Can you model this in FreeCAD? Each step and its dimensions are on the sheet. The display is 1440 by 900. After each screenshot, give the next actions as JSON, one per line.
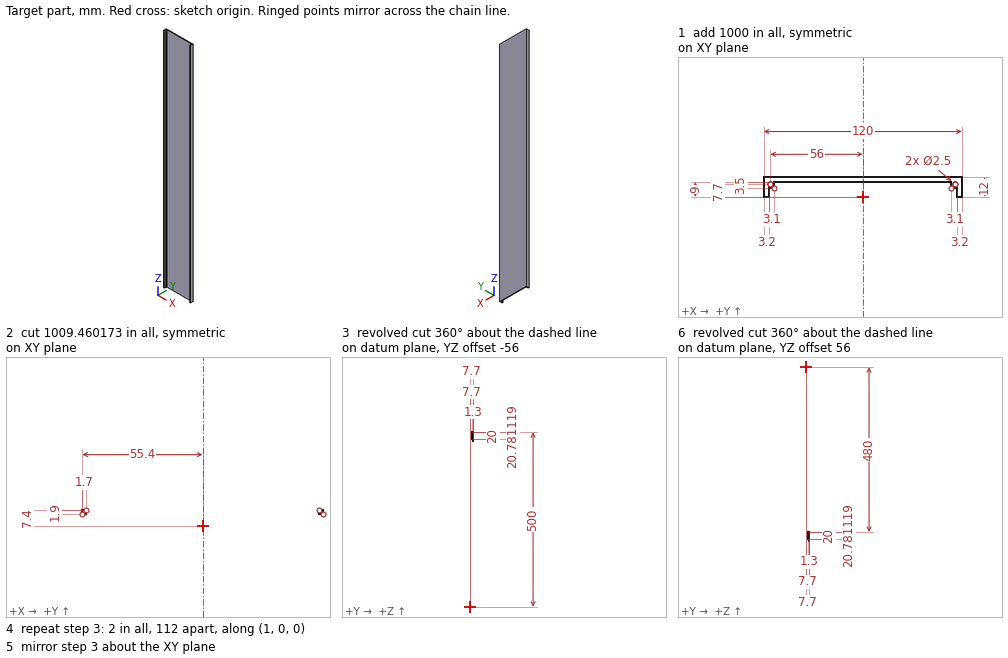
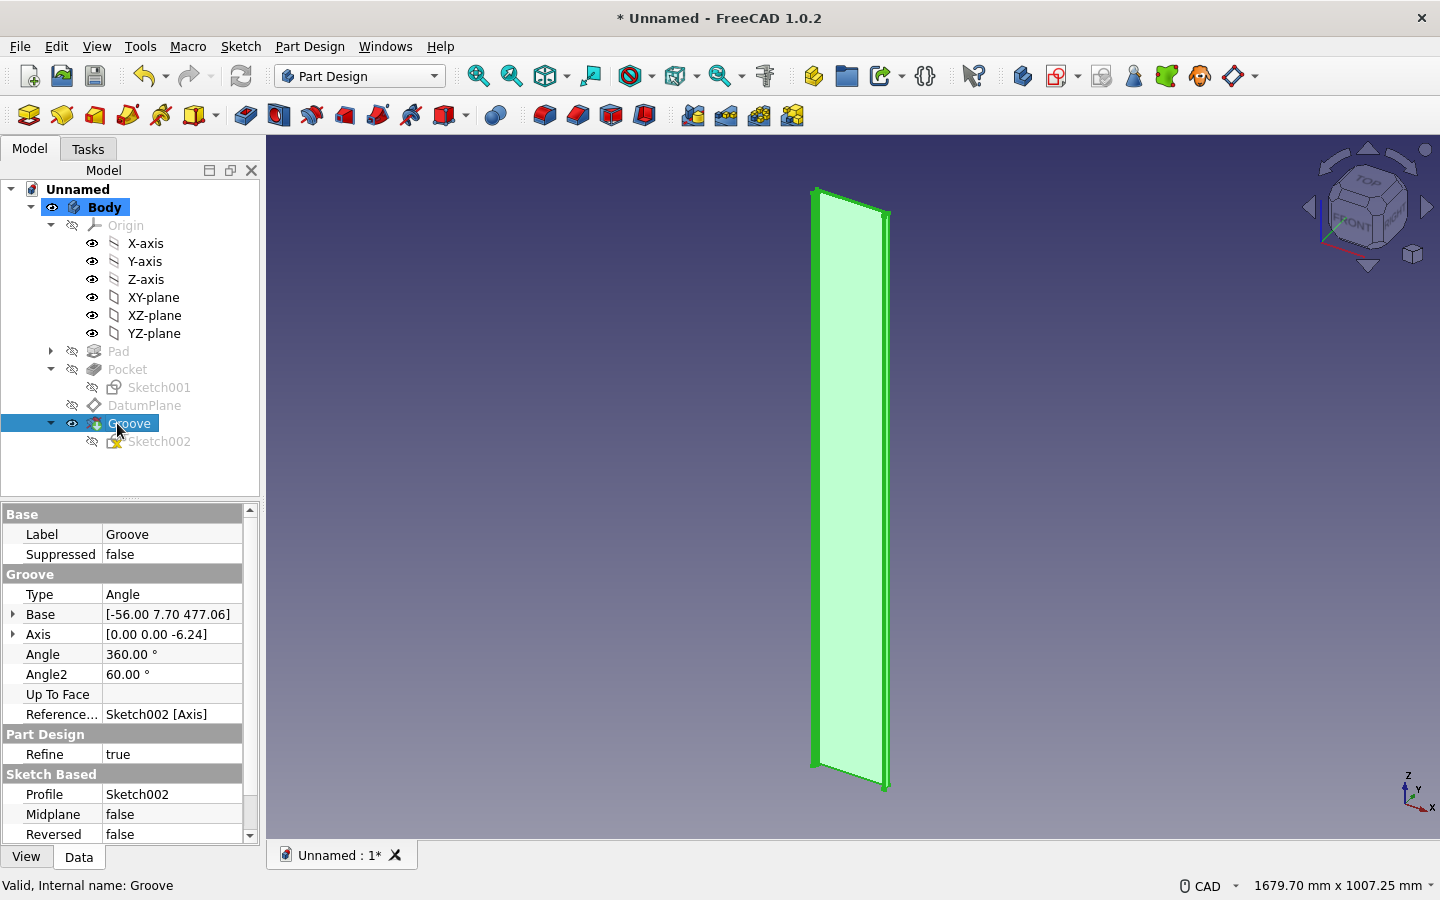
{"action": "left_click", "coordinate": [726, 116]}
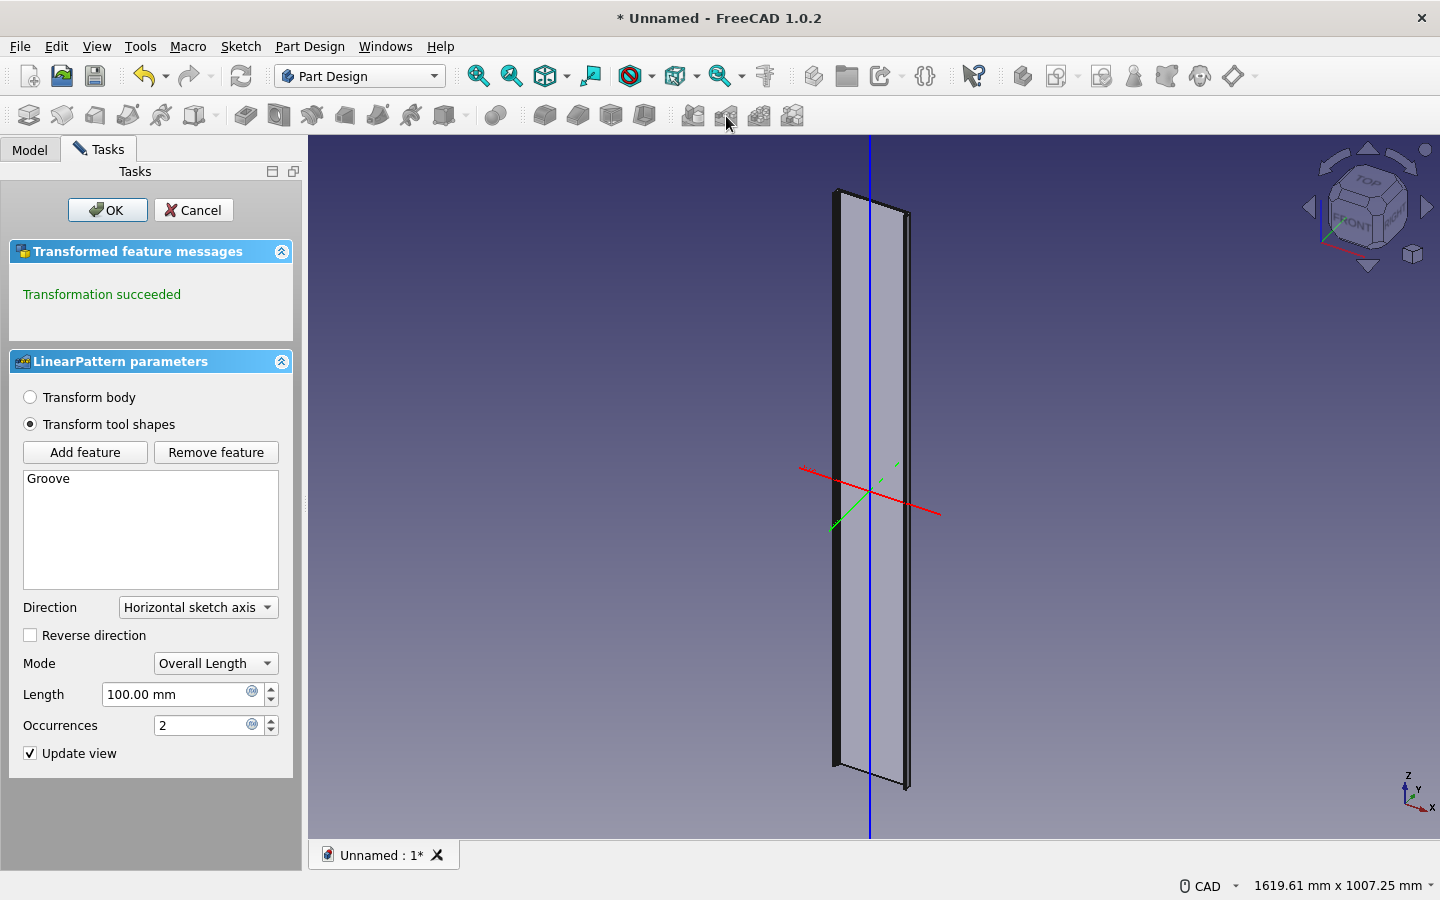
{"action": "left_click", "coordinate": [199, 608]}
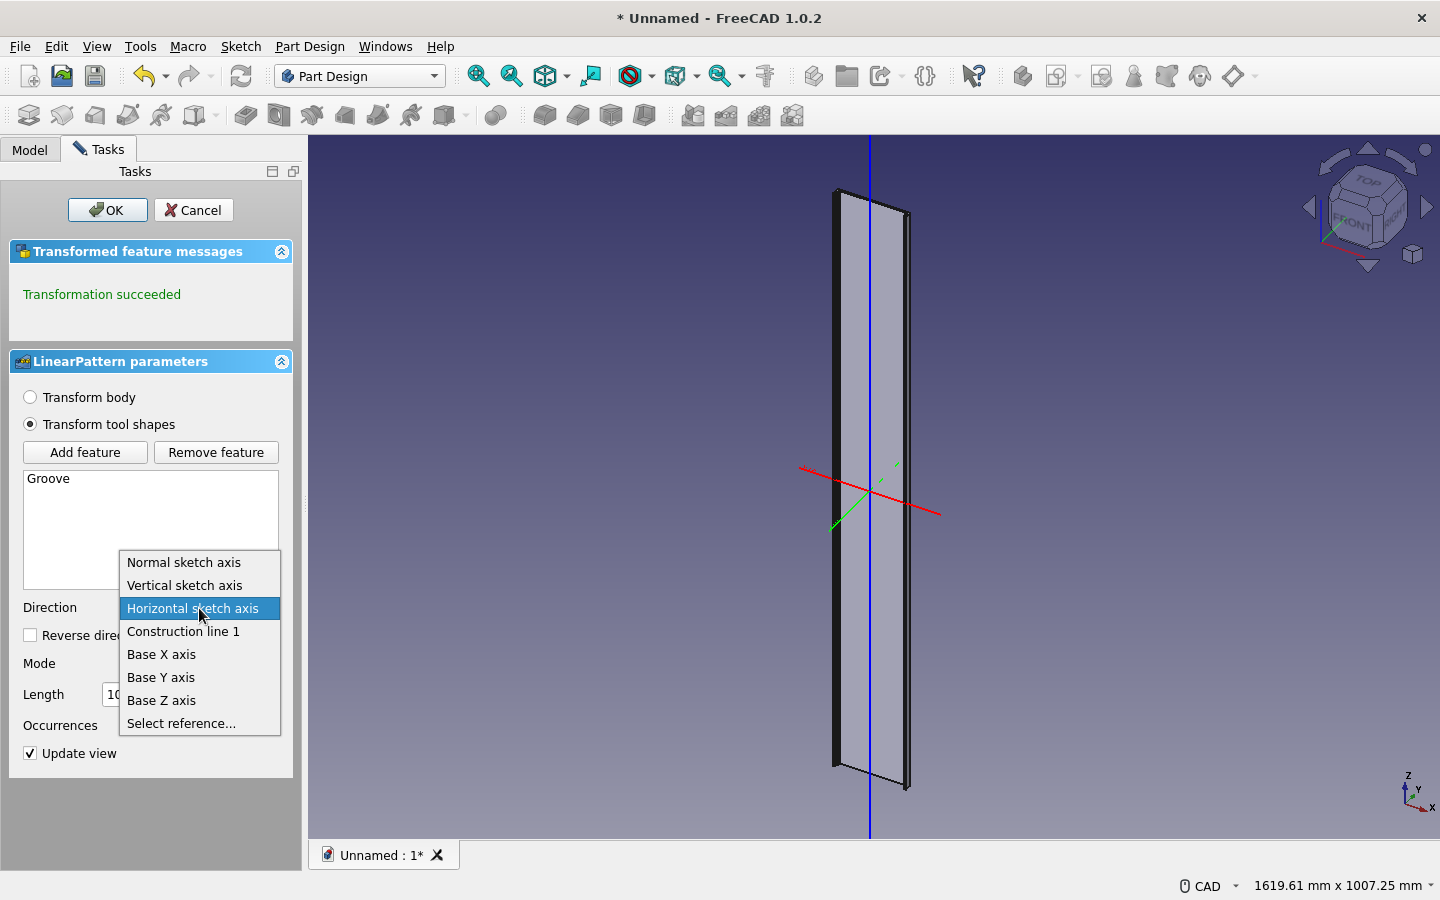
{"action": "left_click", "coordinate": [198, 654]}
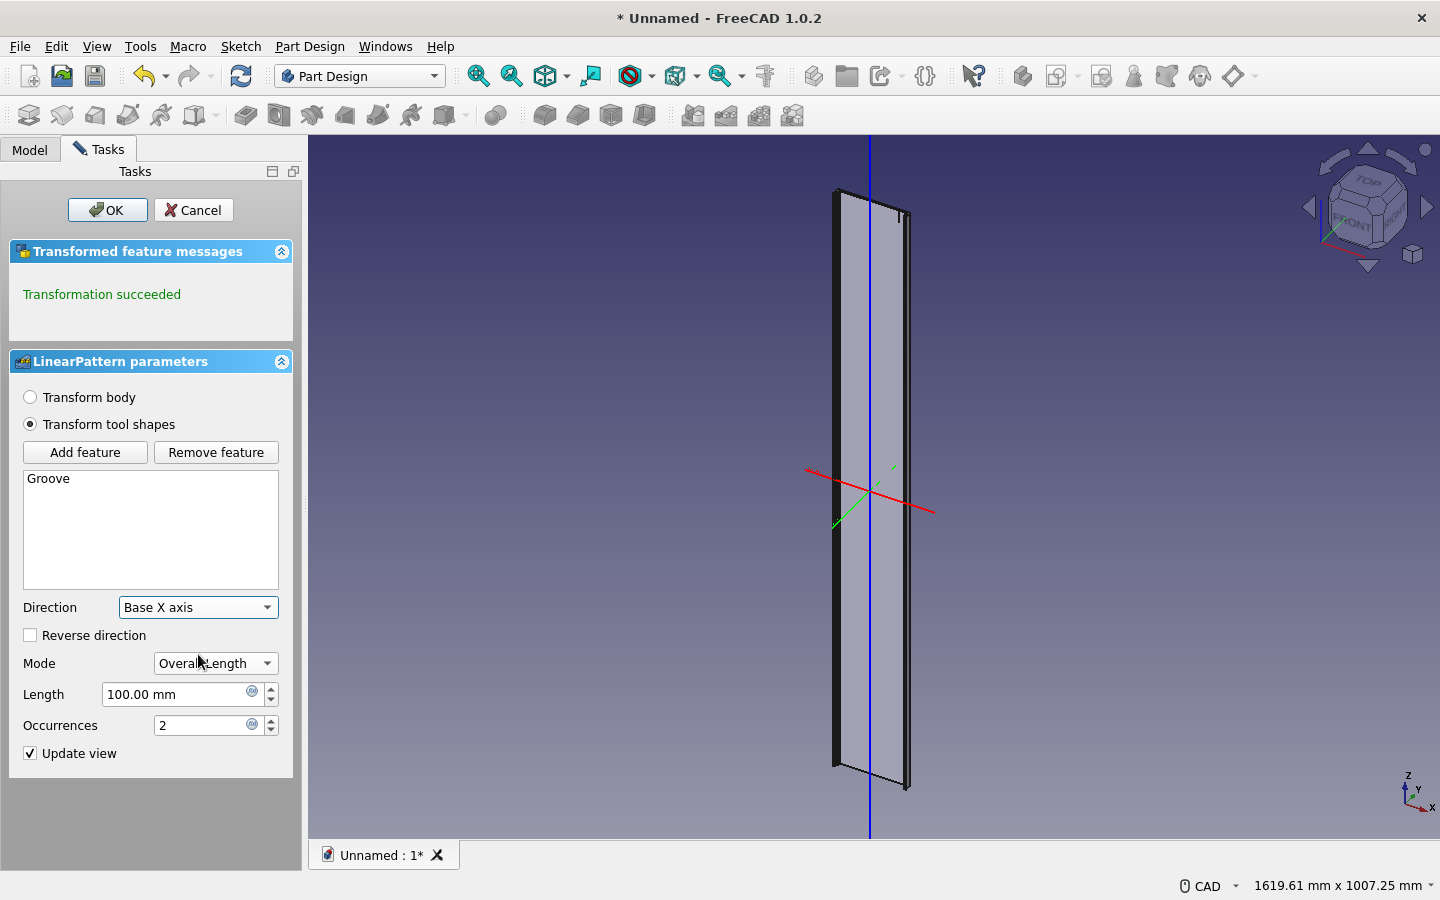
{"action": "left_click", "coordinate": [216, 664]}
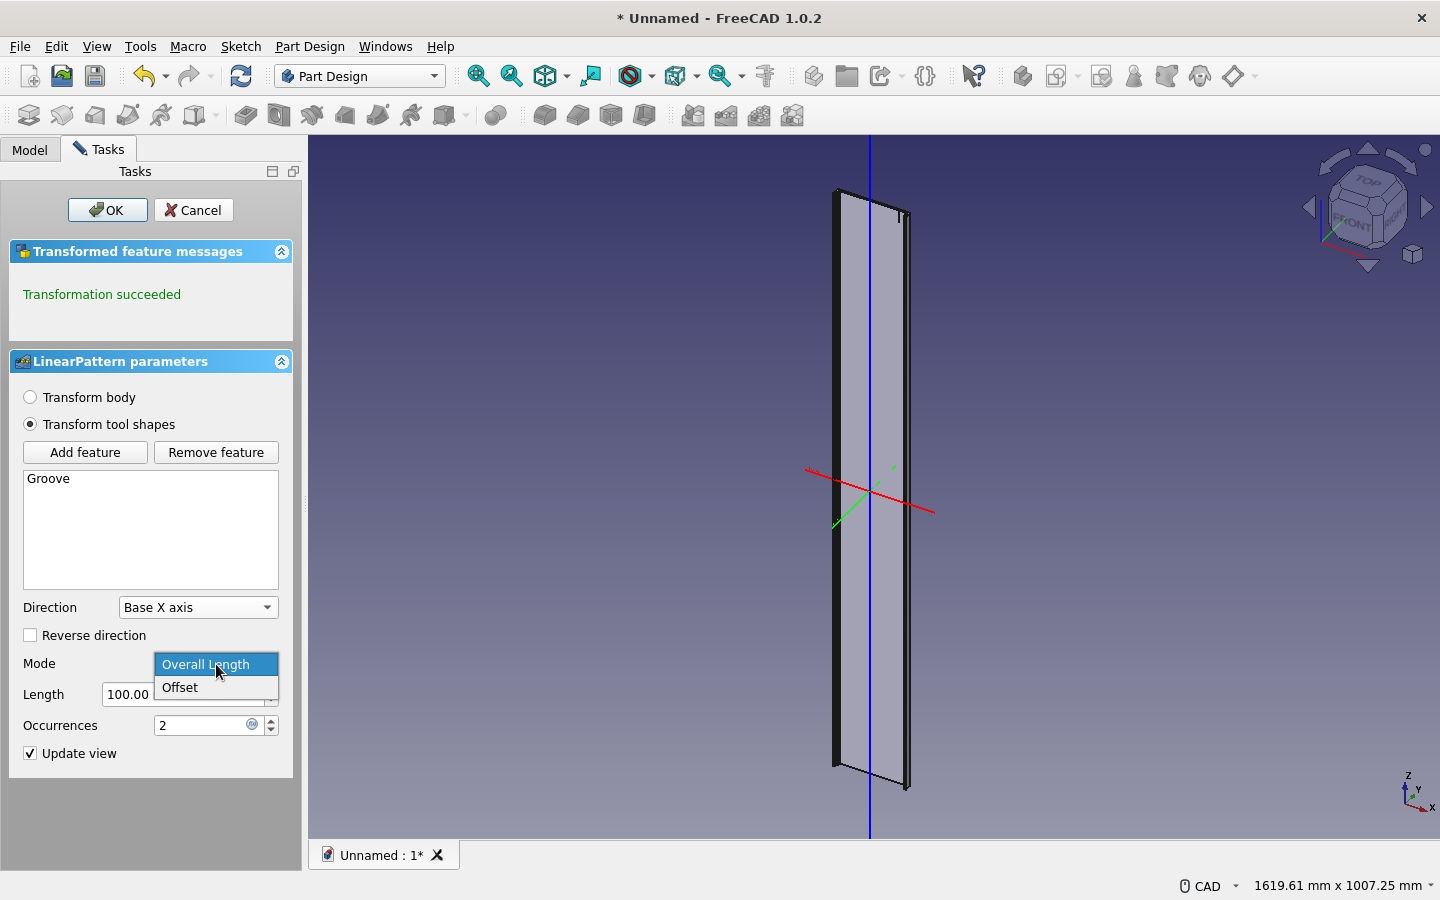
{"action": "left_click", "coordinate": [214, 688]}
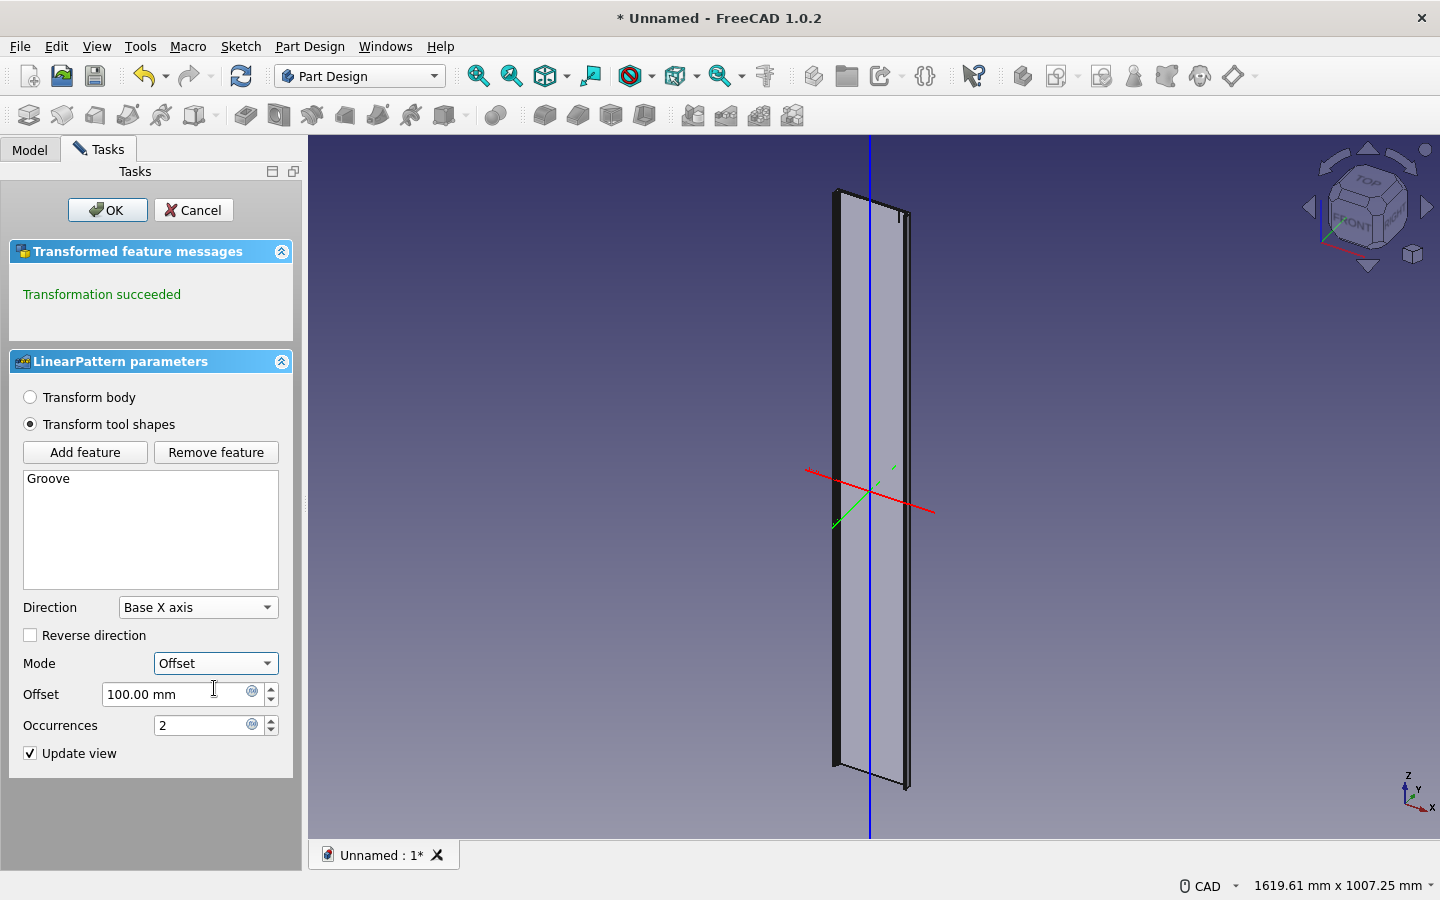
{"action": "triple_click", "coordinate": [184, 694]}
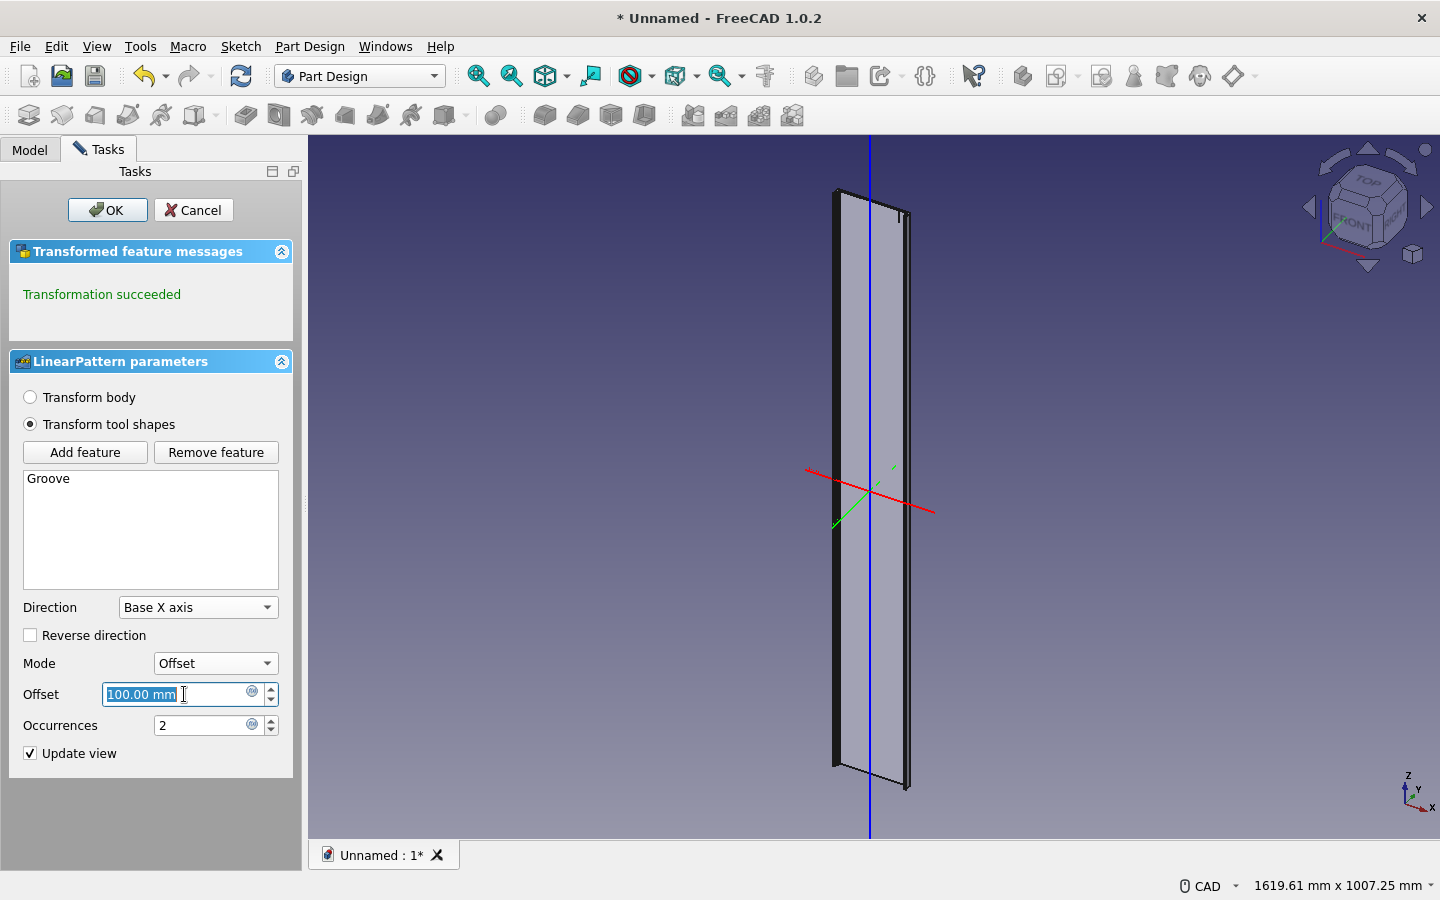
{"action": "type", "text": "112"}
{"action": "key", "text": "Tab"}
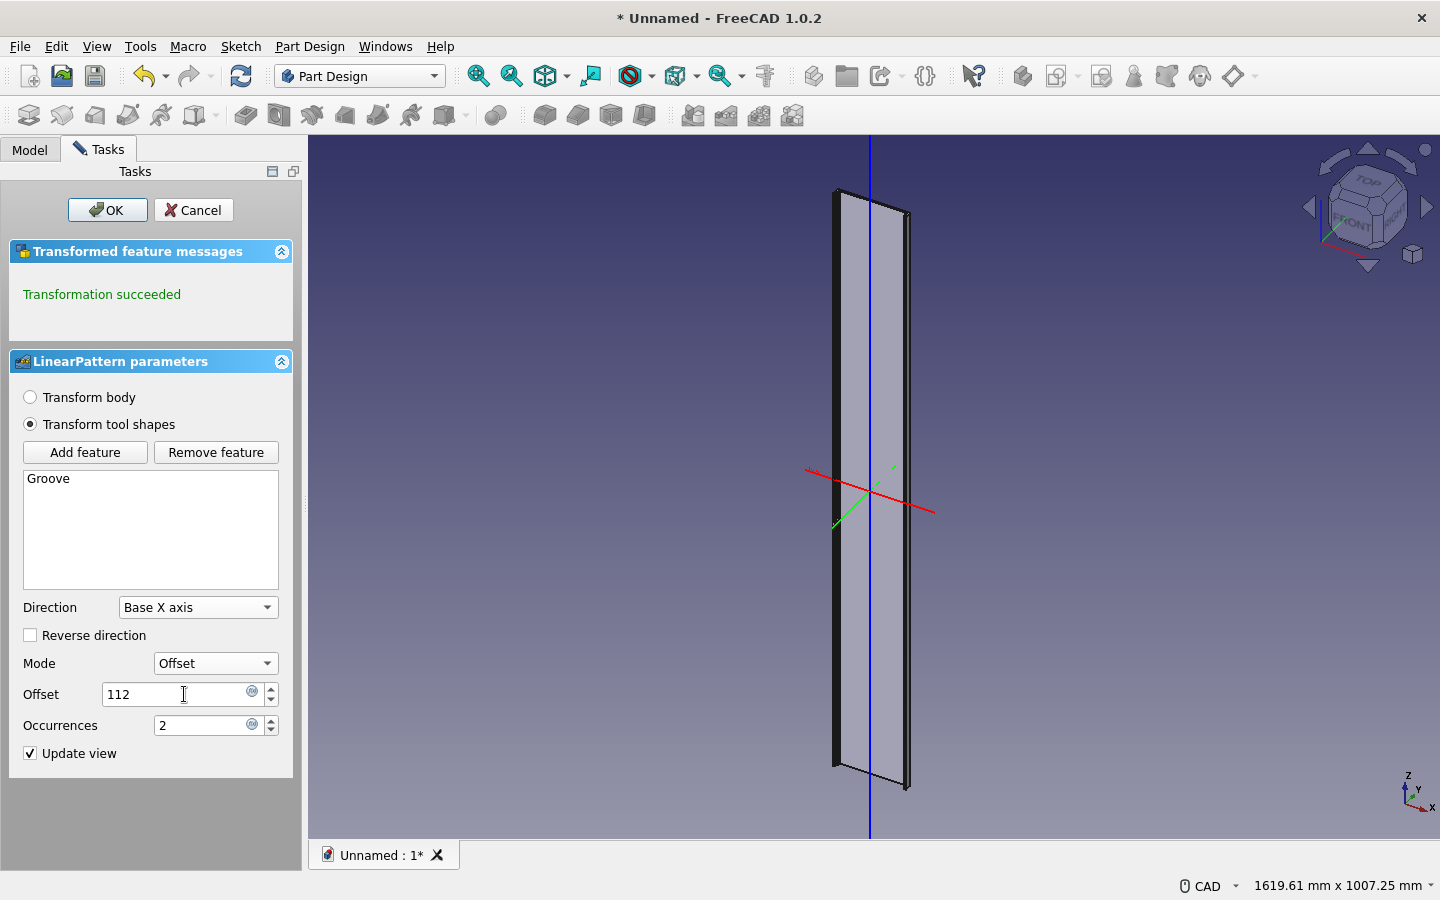
{"action": "triple_click", "coordinate": [210, 726]}